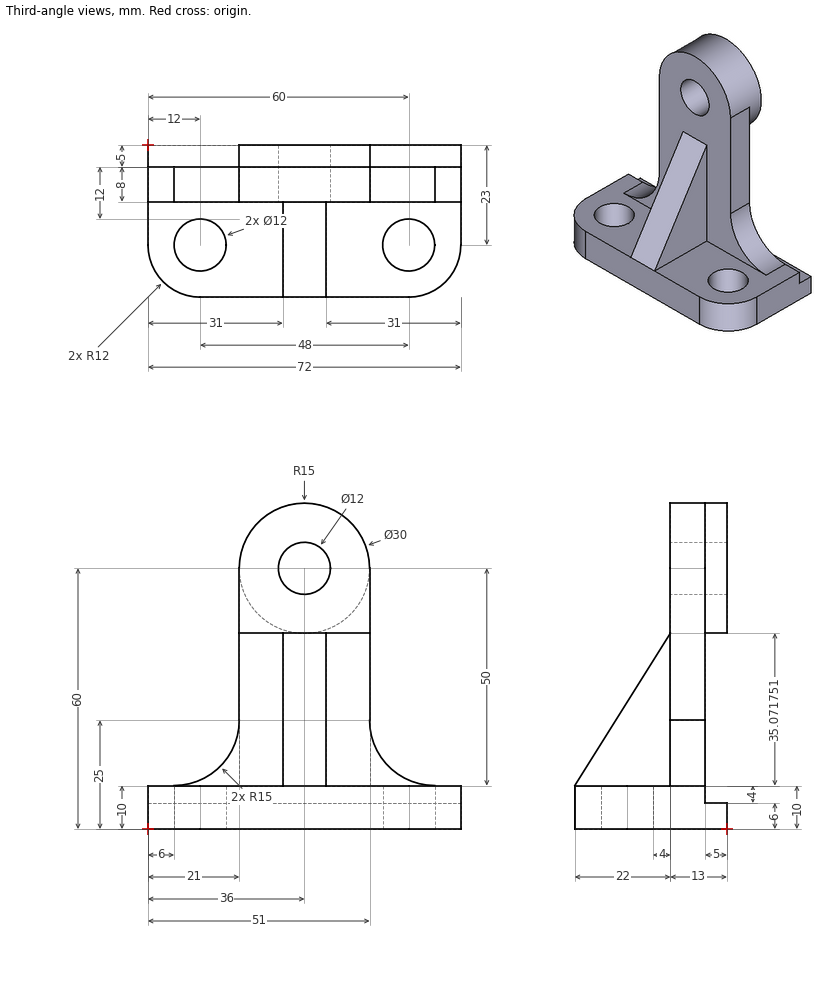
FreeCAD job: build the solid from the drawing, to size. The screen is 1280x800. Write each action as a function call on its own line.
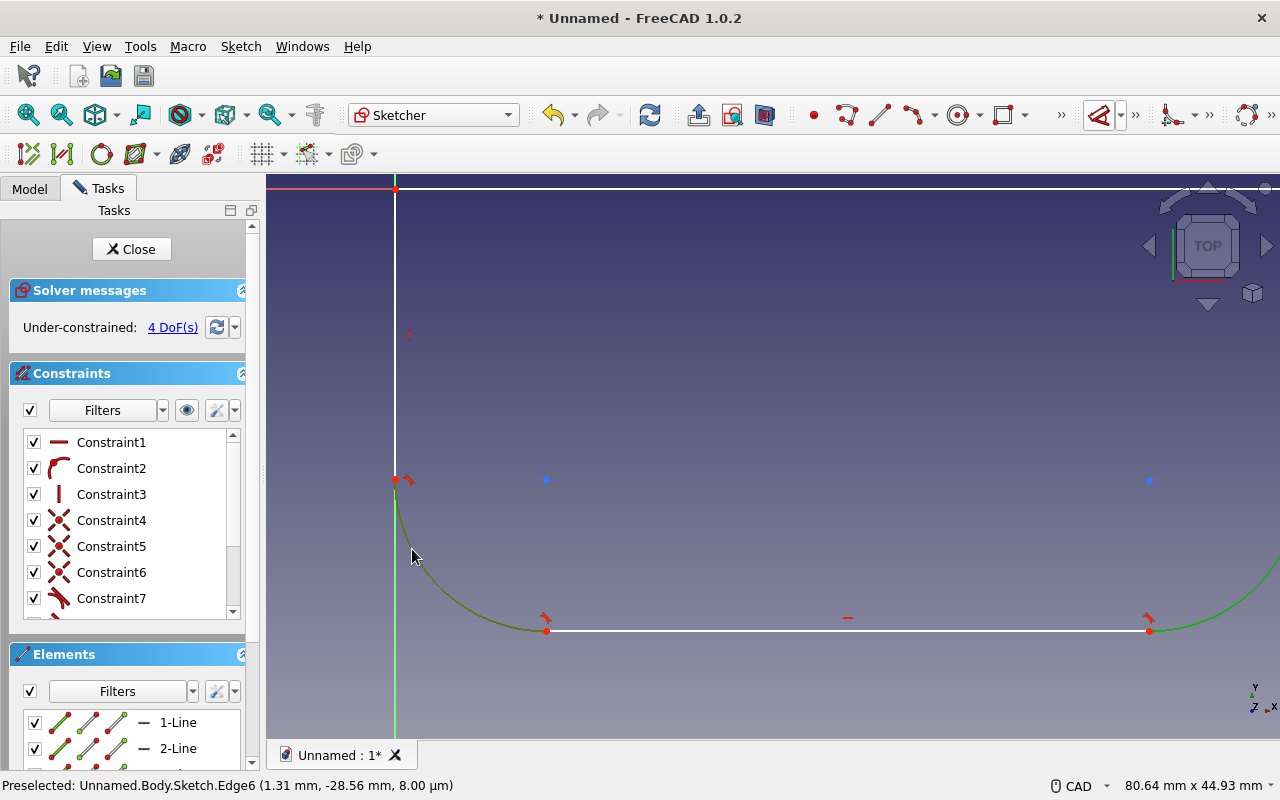
key(e)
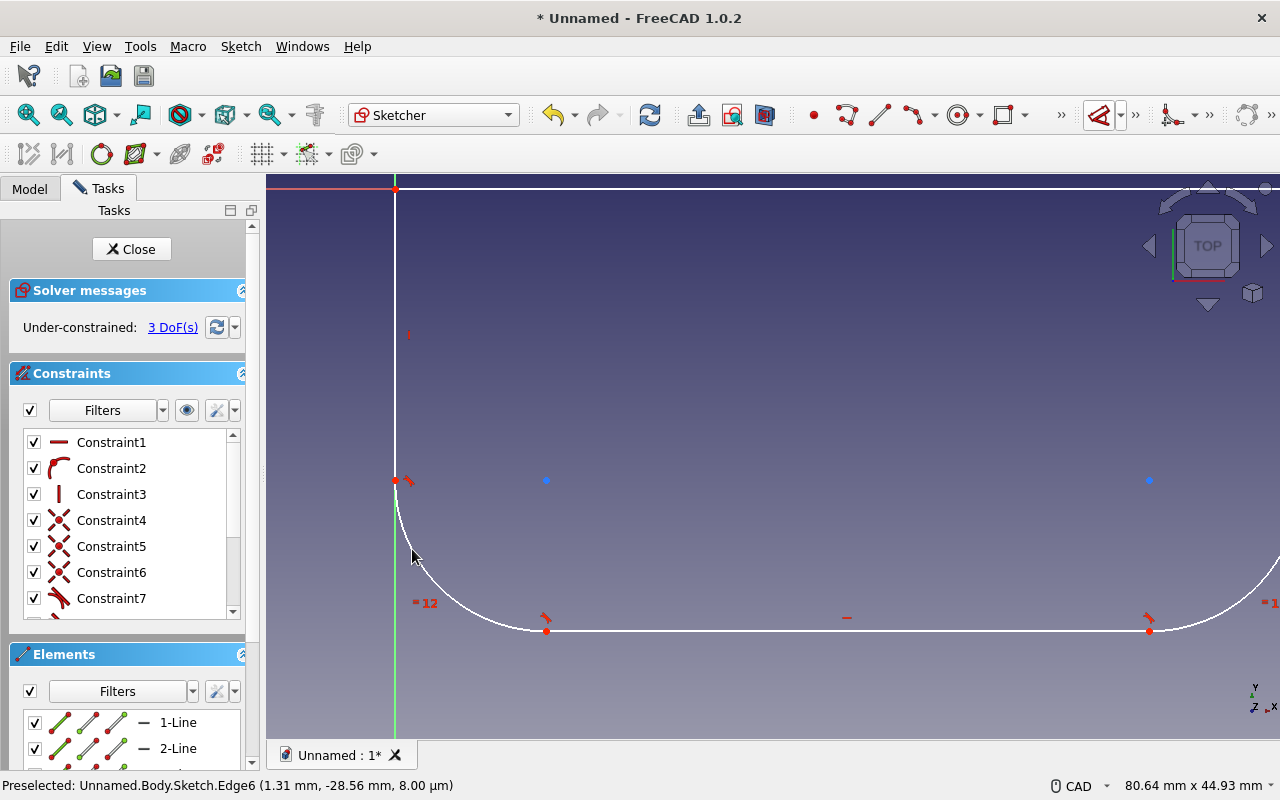
click(1098, 116)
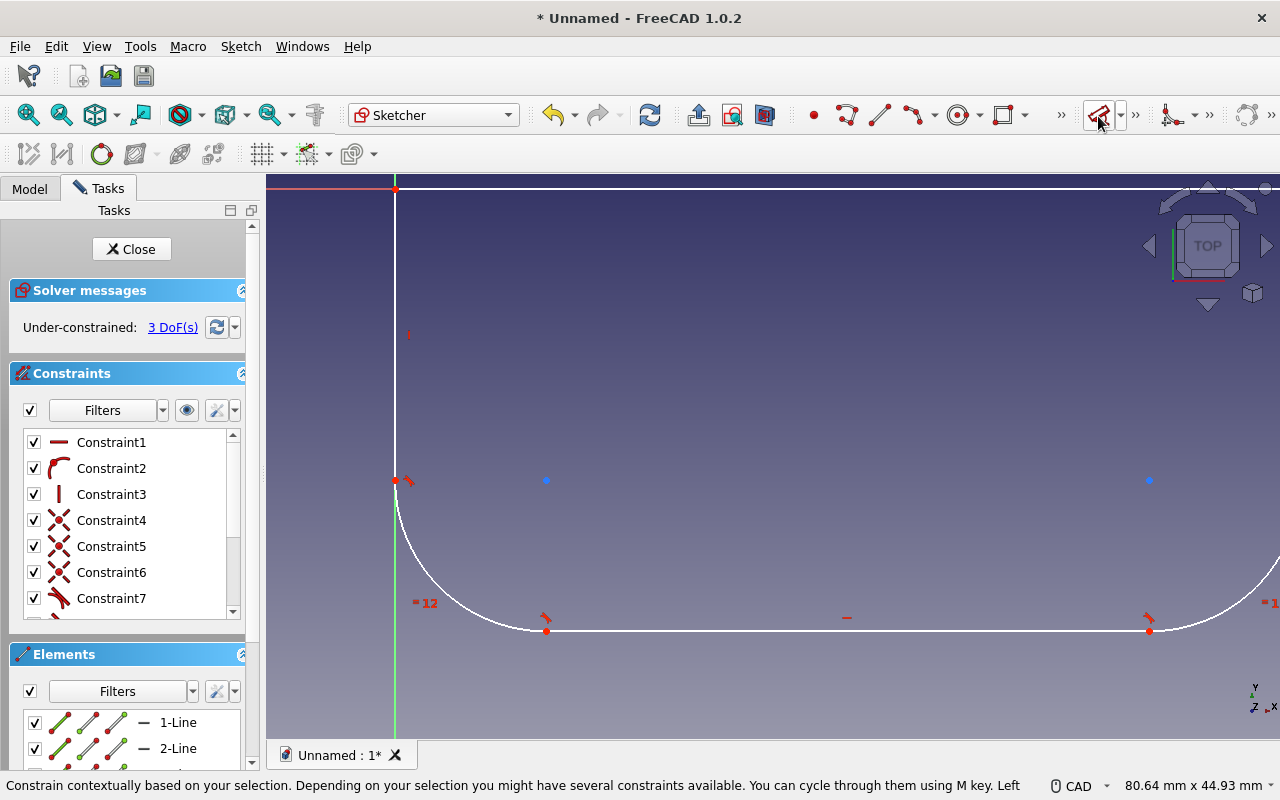
scroll(413, 552, down, 2)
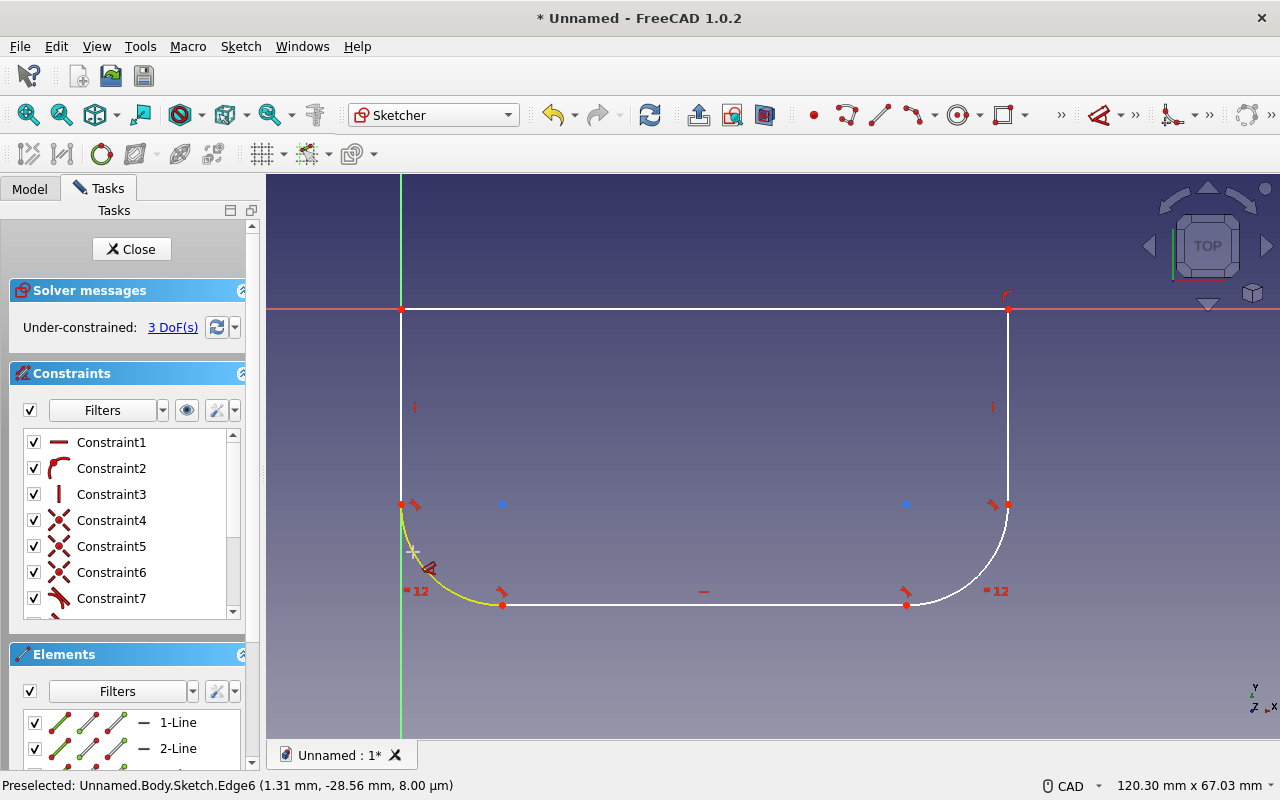
click(953, 594)
click(968, 622)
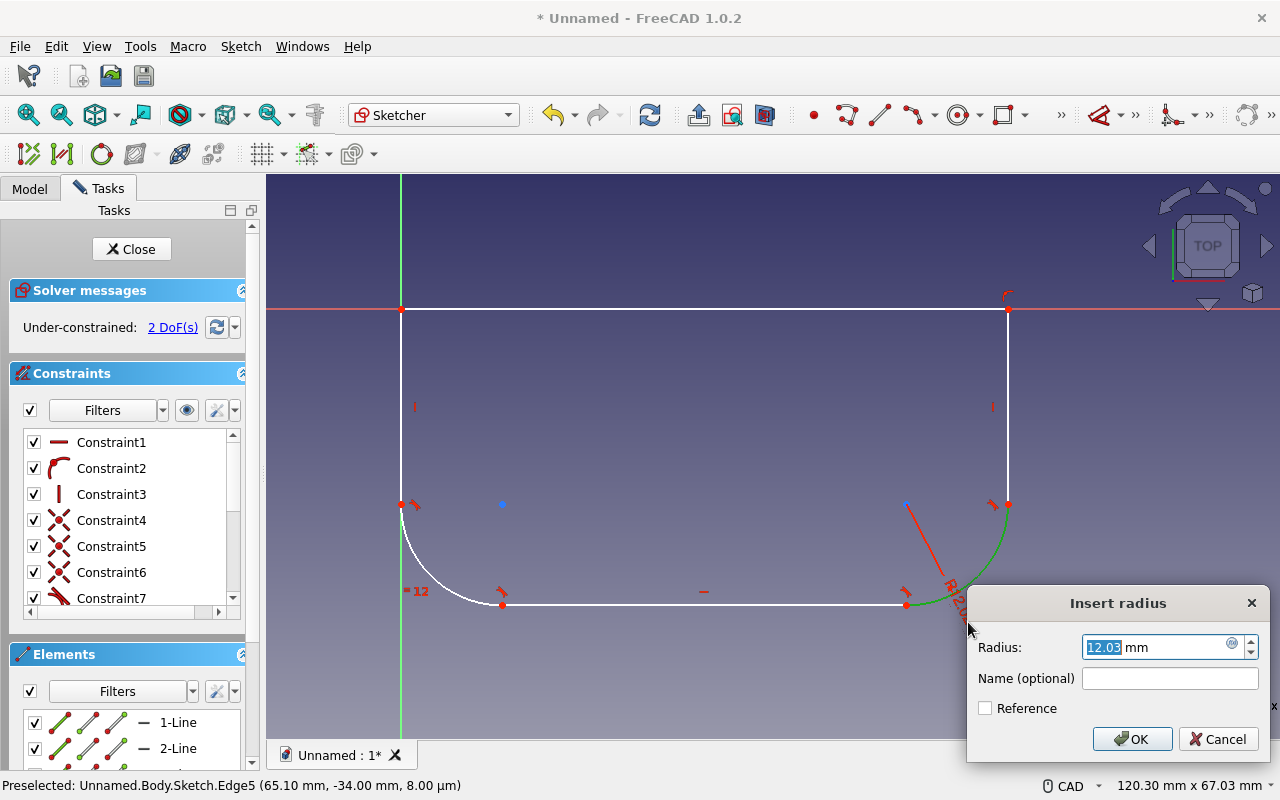
text(12)
key(Return)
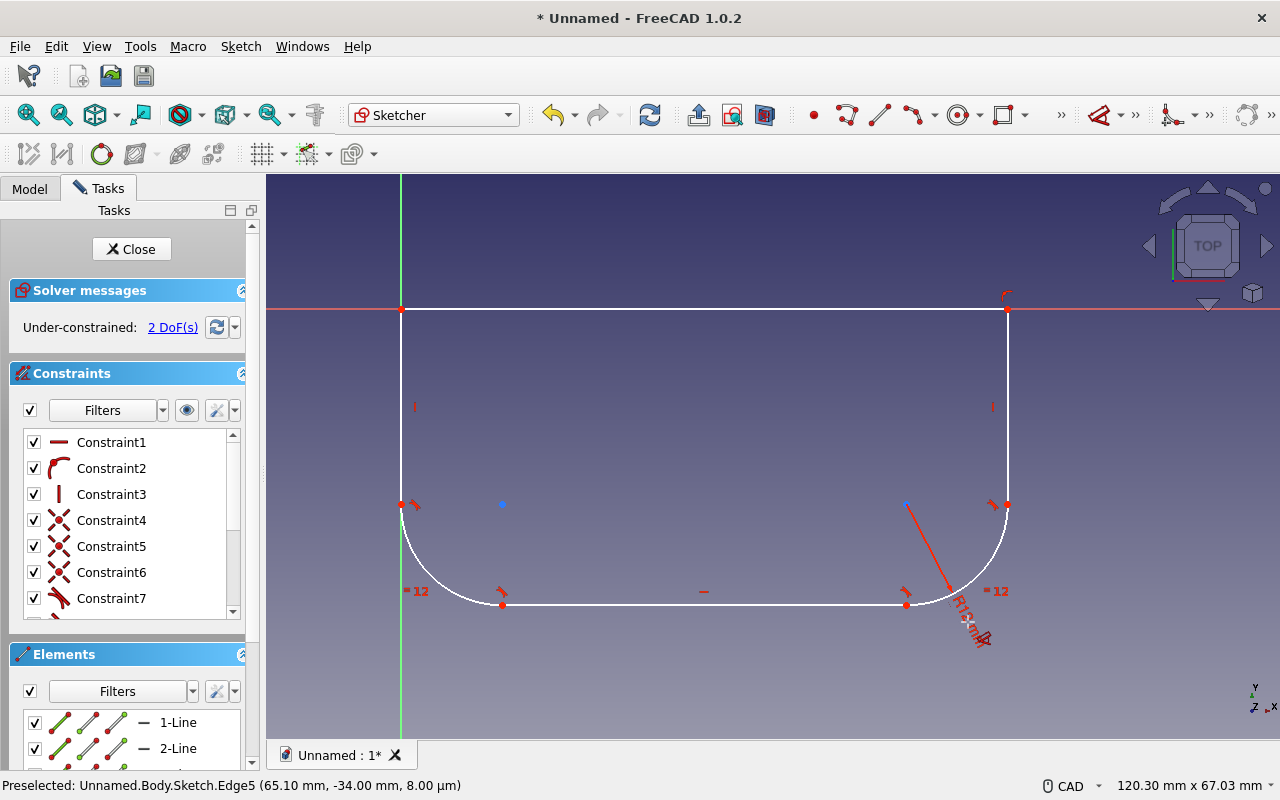
click(624, 605)
click(704, 639)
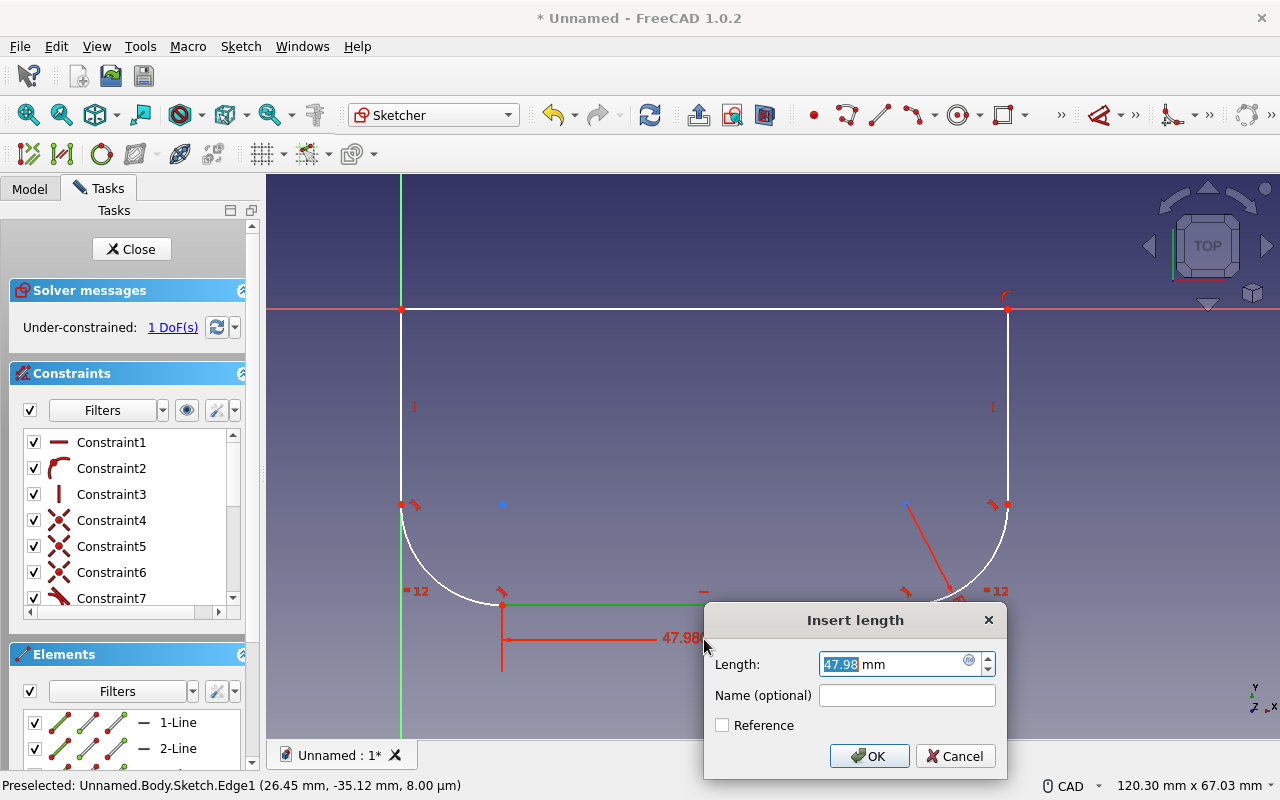
text(48)
key(Return)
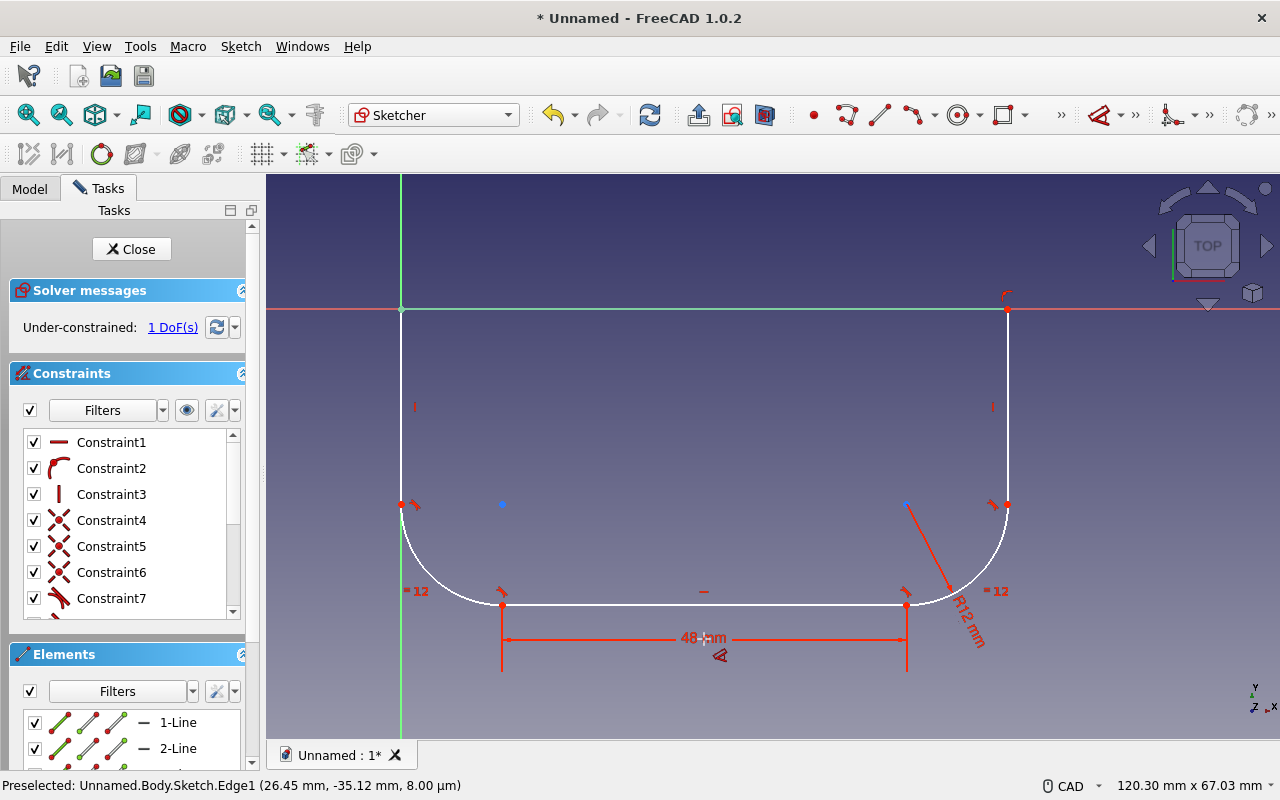
click(1008, 446)
click(1042, 407)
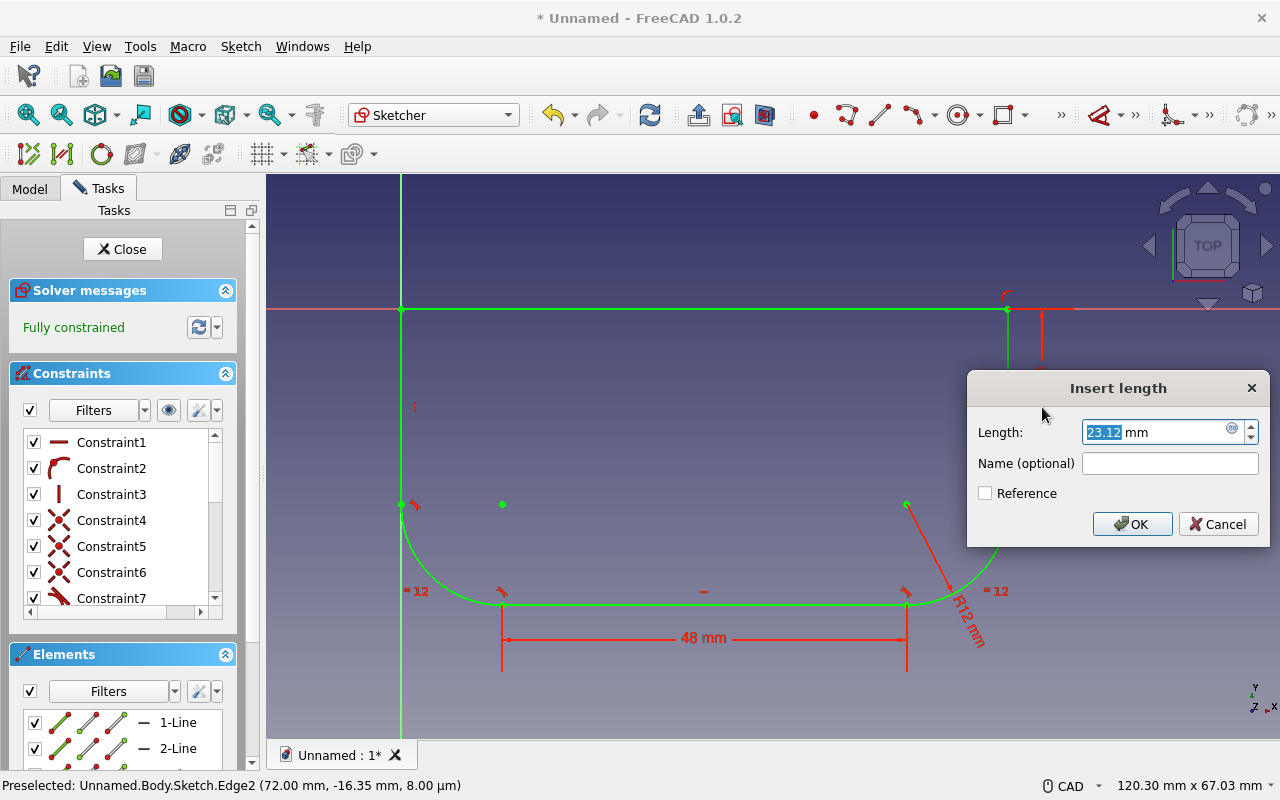
text(23)
key(Return)
key(Escape)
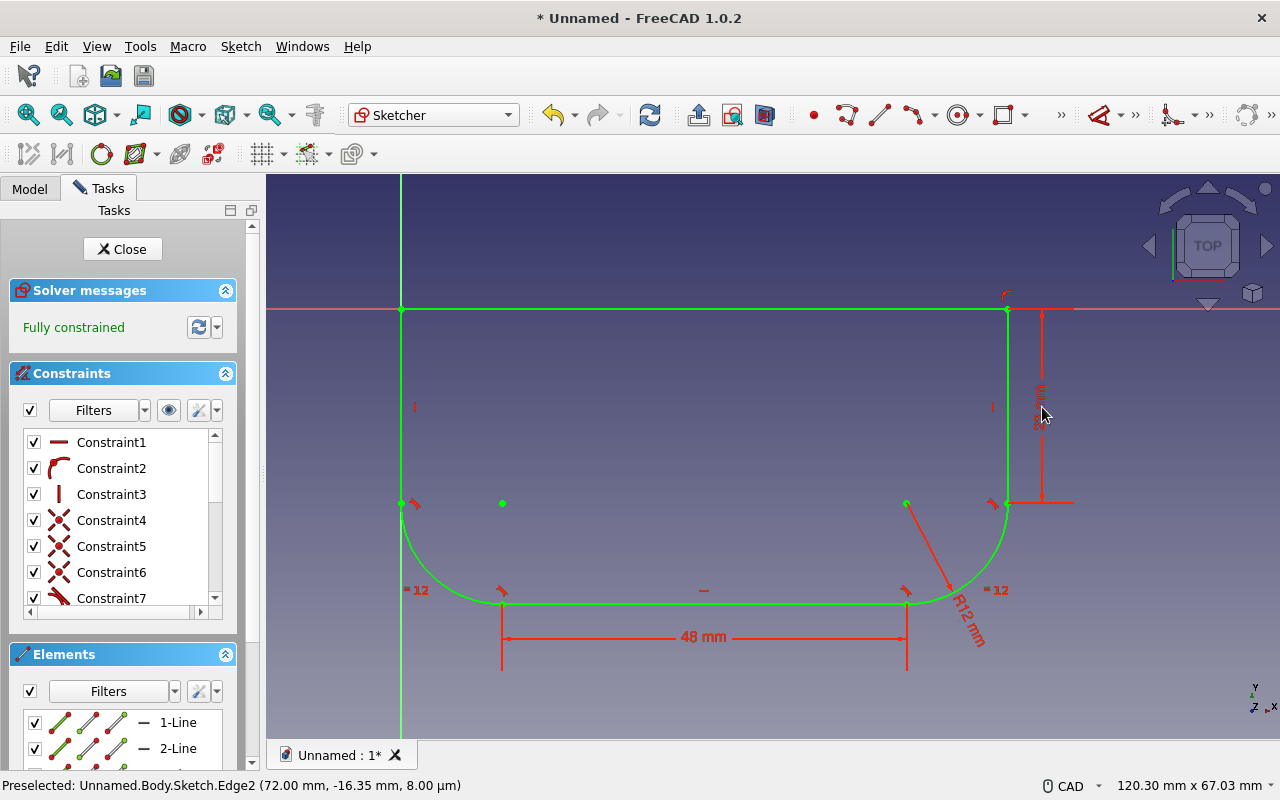
click(123, 249)